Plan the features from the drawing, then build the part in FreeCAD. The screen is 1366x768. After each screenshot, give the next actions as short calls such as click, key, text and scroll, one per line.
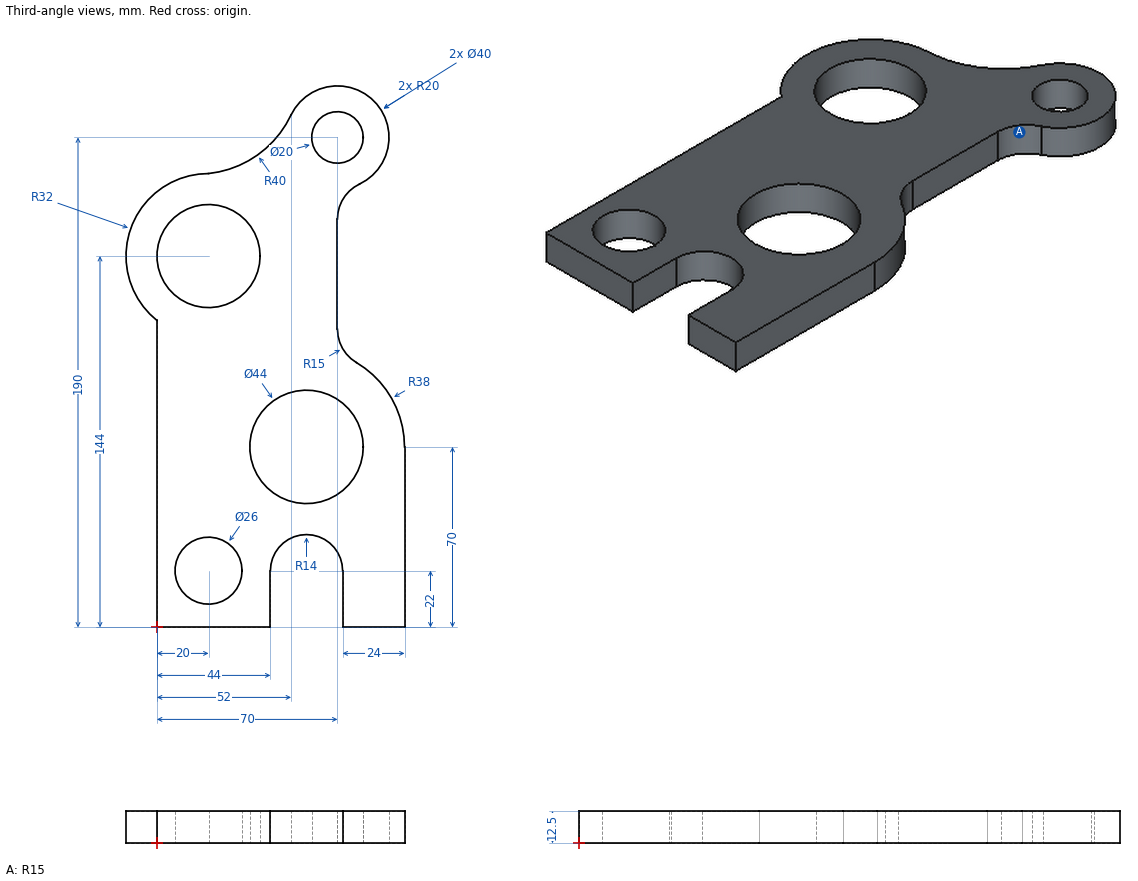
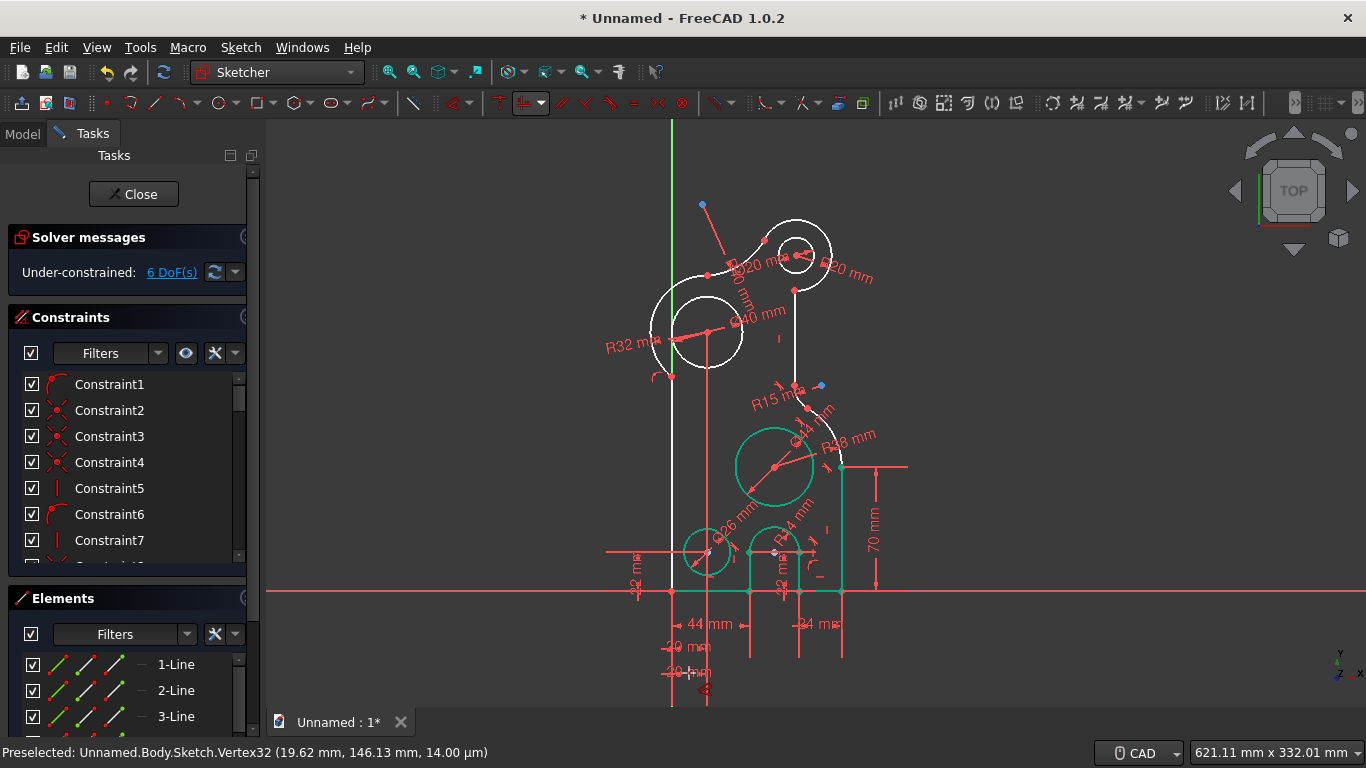
click(796, 255)
click(734, 221)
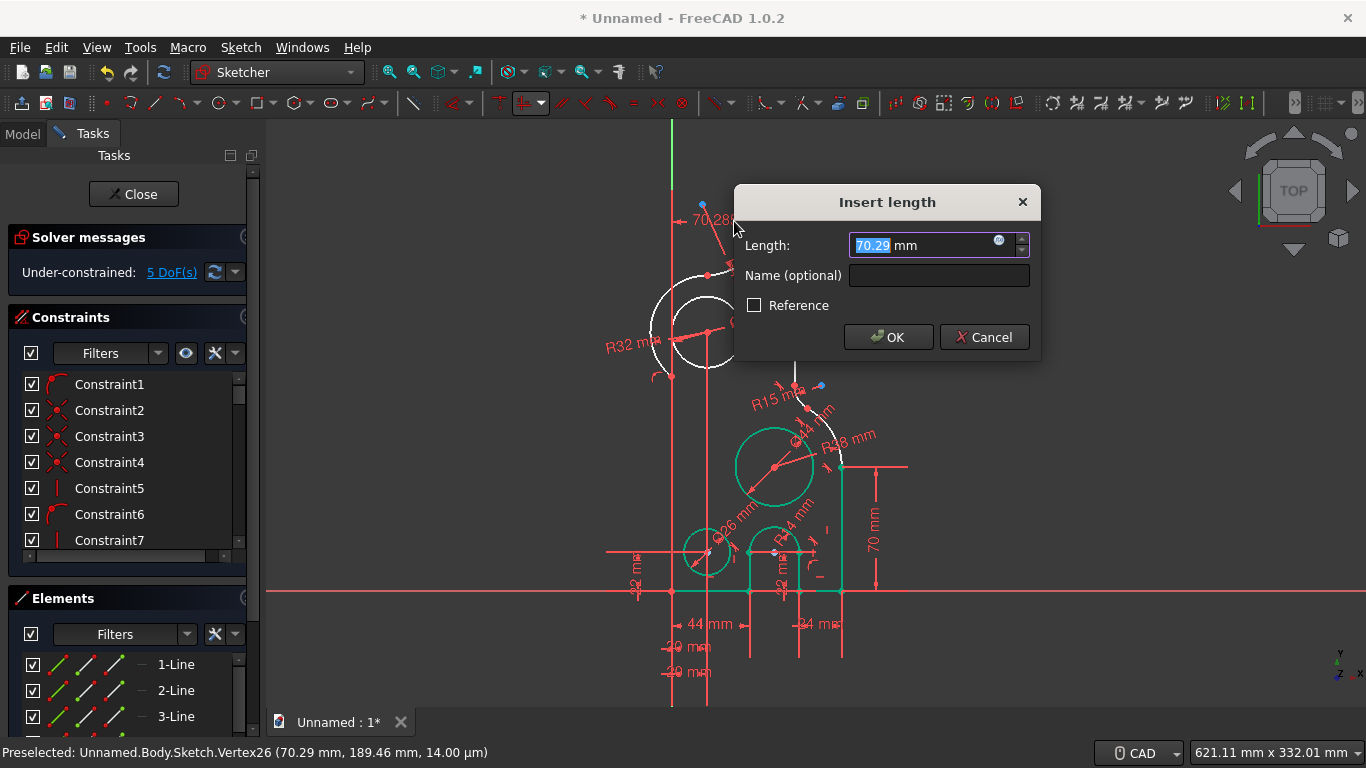
text(70)
key(Return)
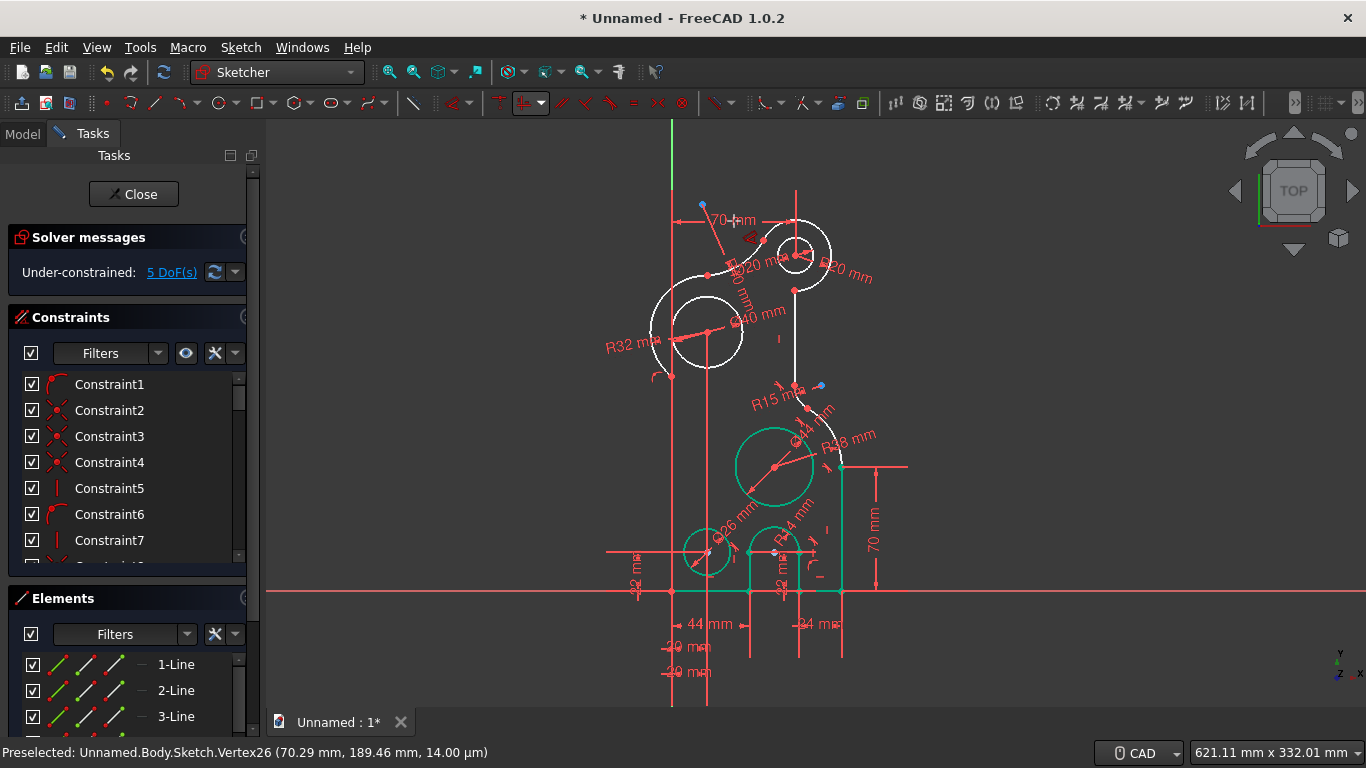
click(795, 386)
click(705, 352)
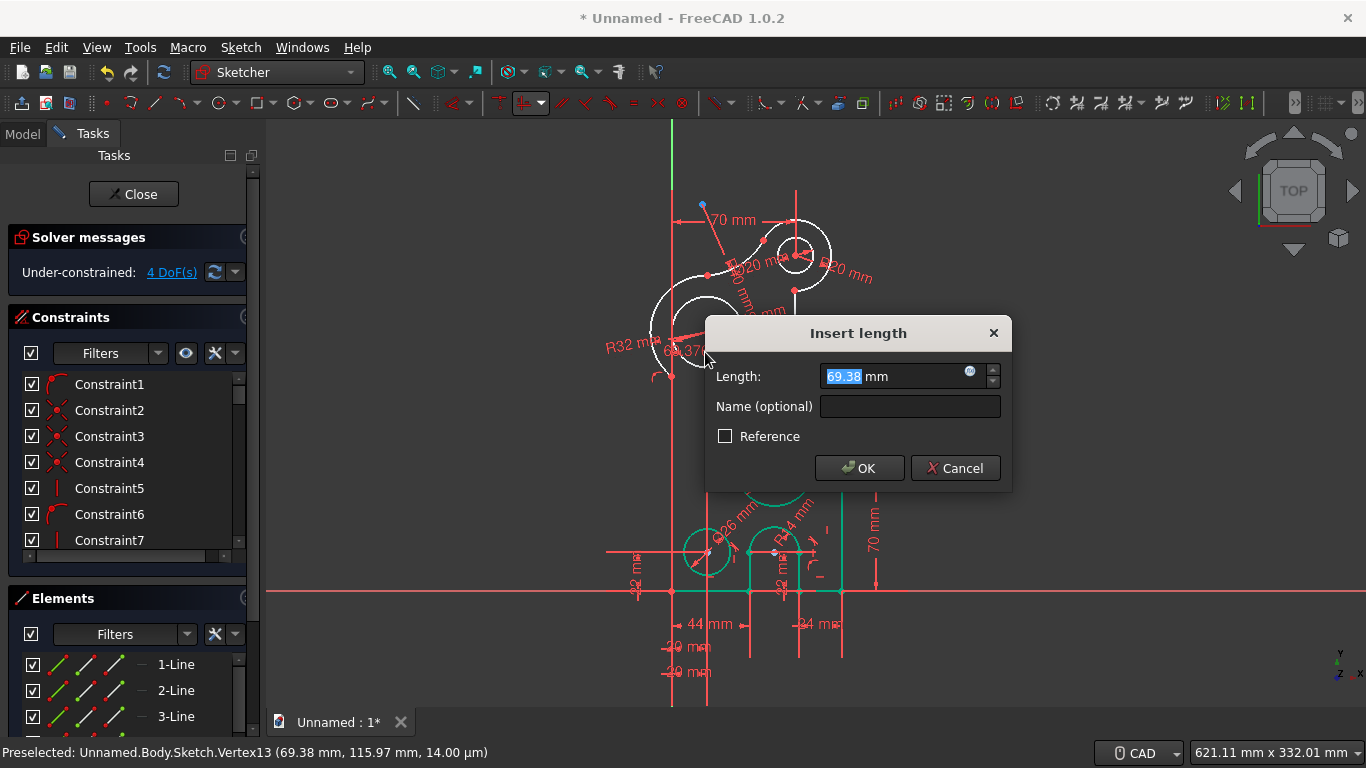
text(70)
key(Return)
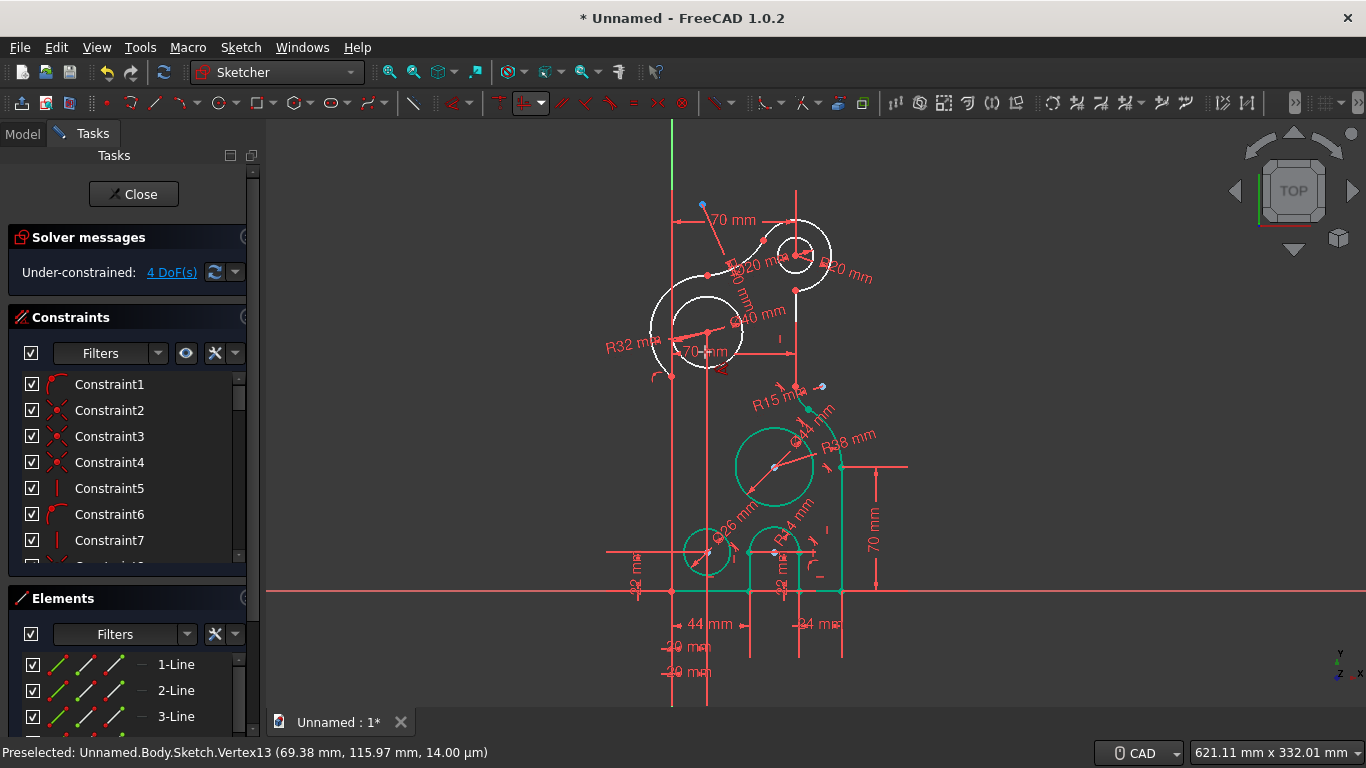
click(764, 240)
click(718, 182)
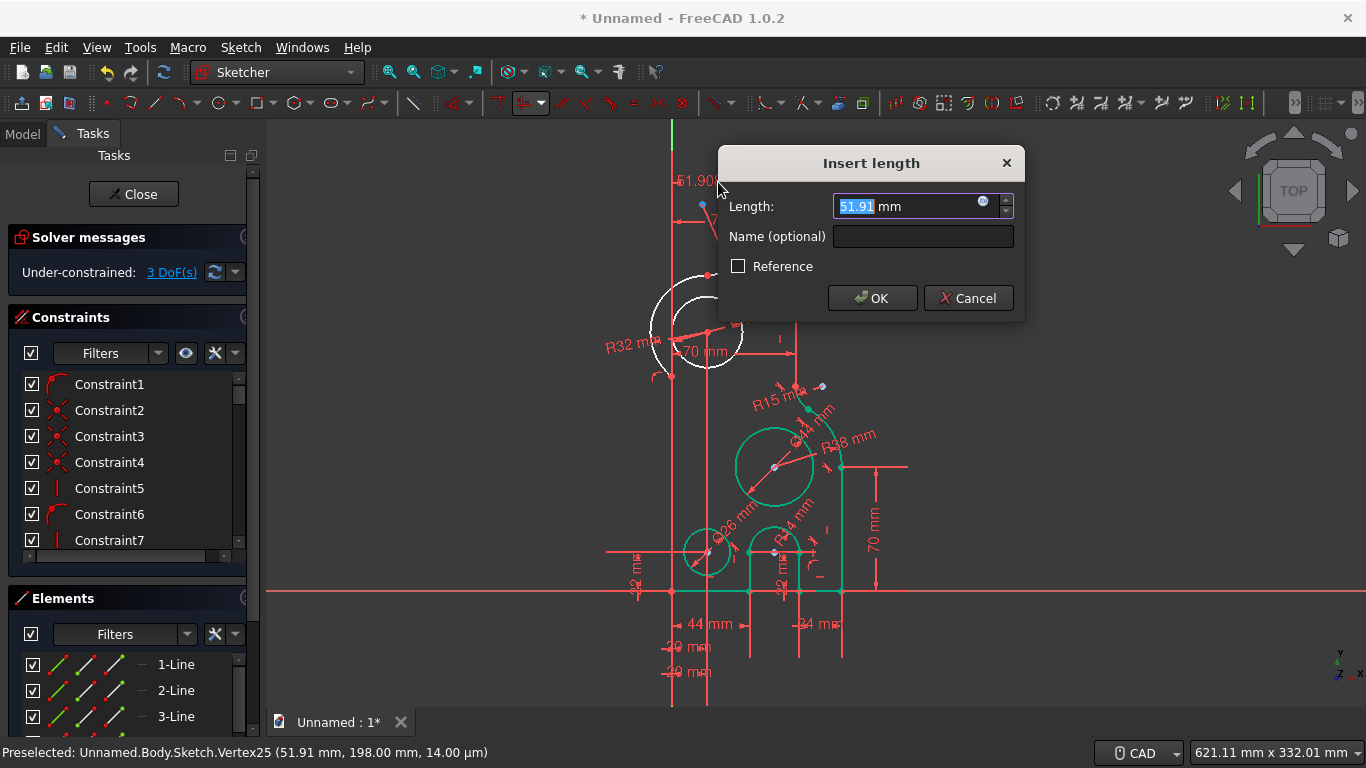
text(52)
key(Return)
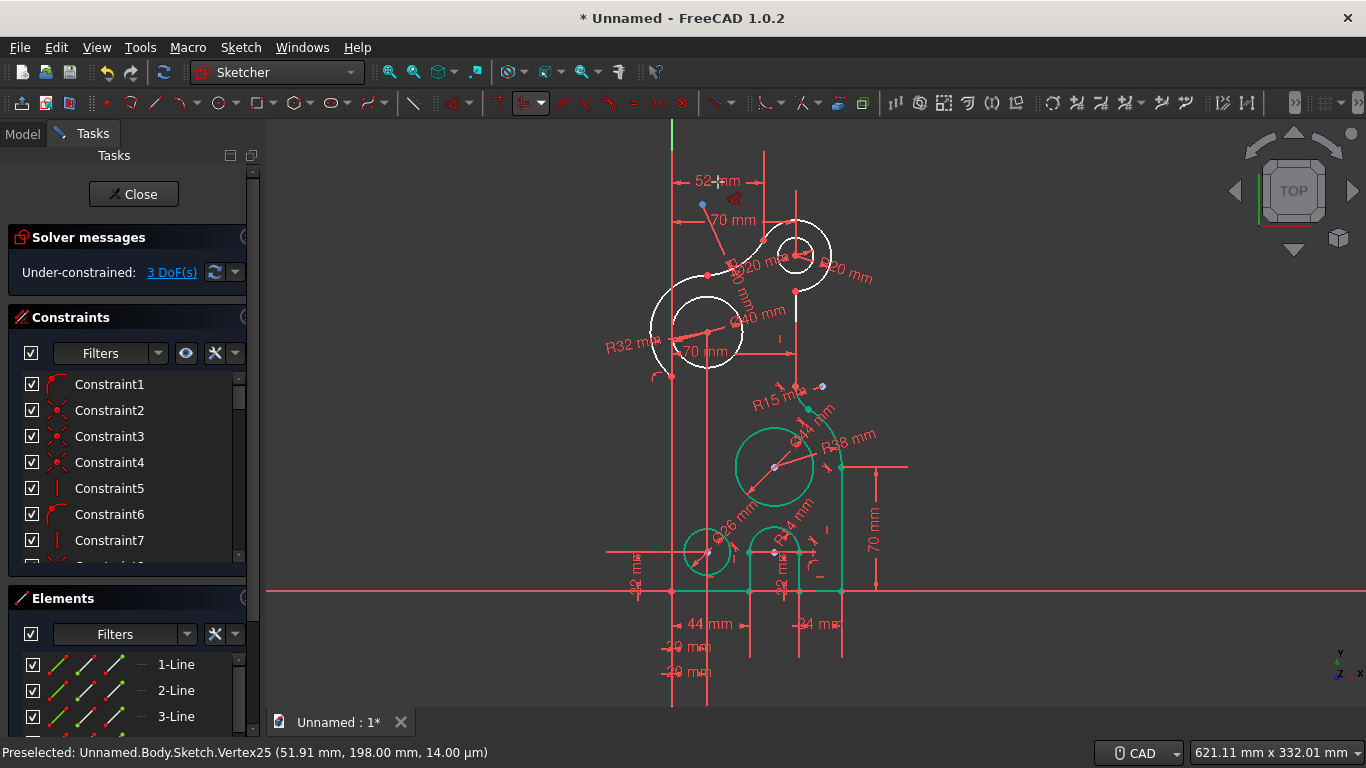
click(707, 276)
click(689, 242)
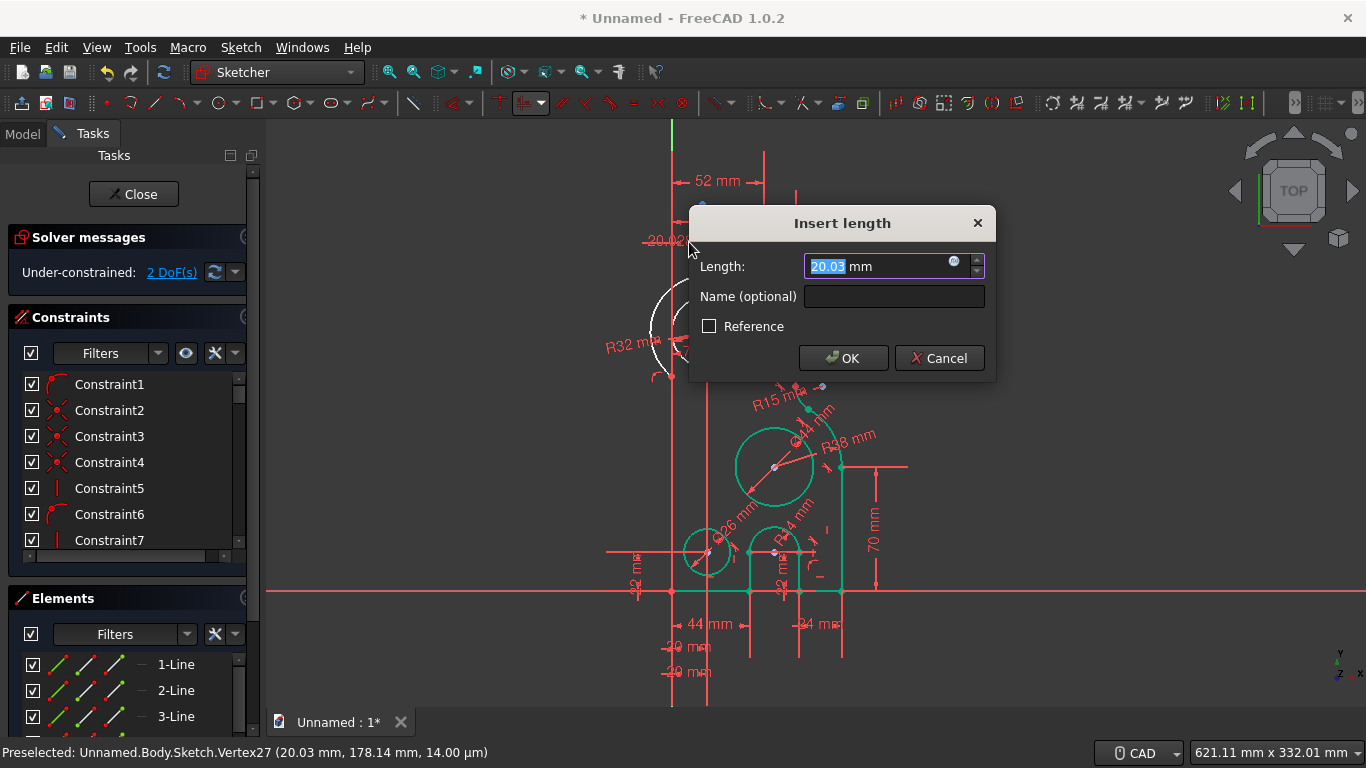
text(20)
key(Return)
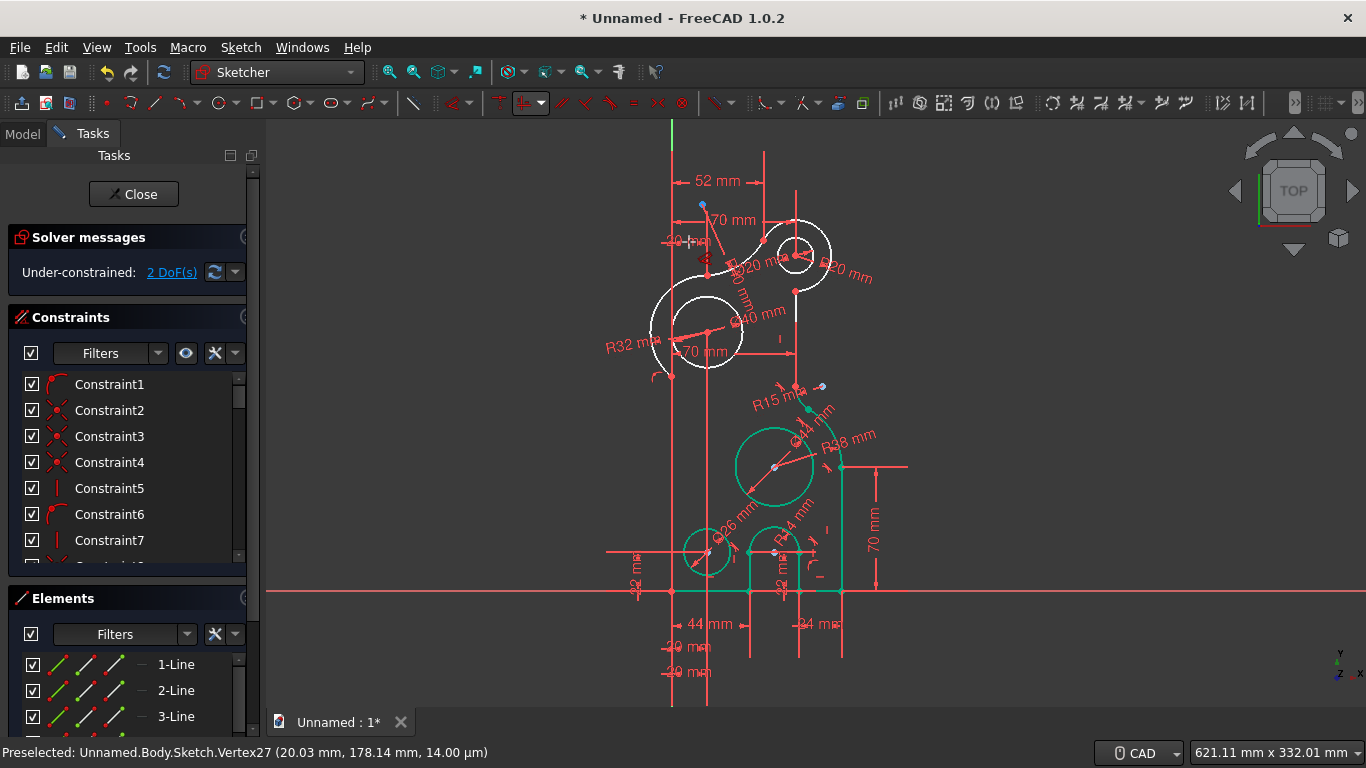
click(707, 332)
click(638, 462)